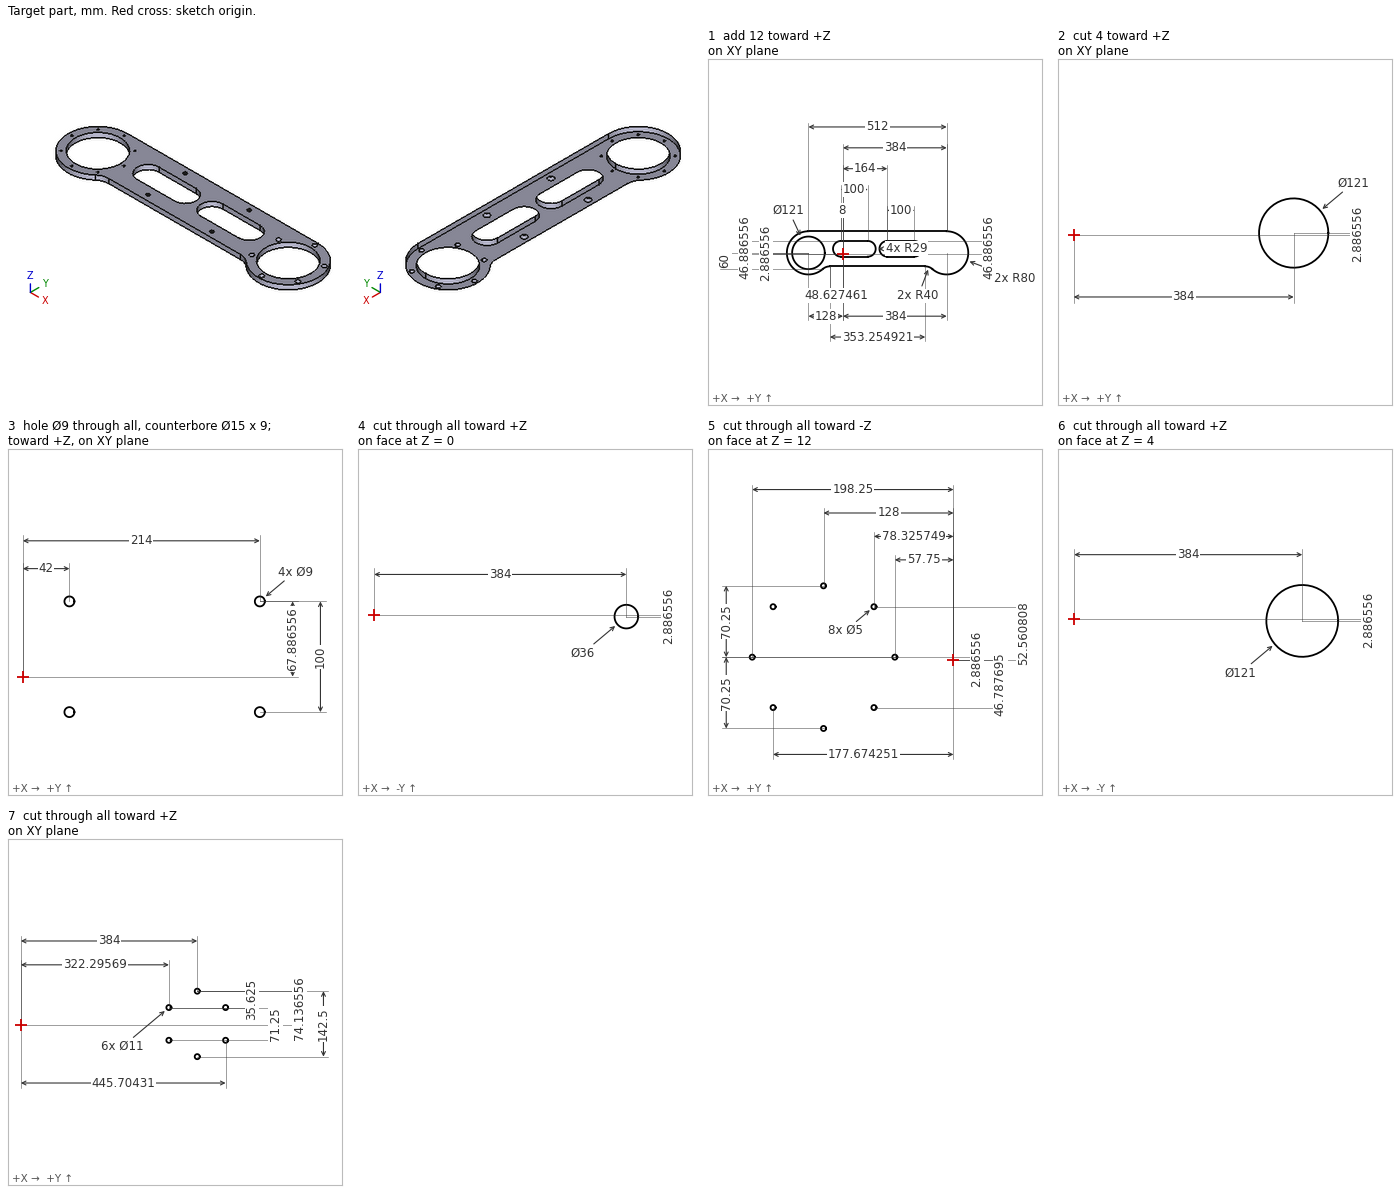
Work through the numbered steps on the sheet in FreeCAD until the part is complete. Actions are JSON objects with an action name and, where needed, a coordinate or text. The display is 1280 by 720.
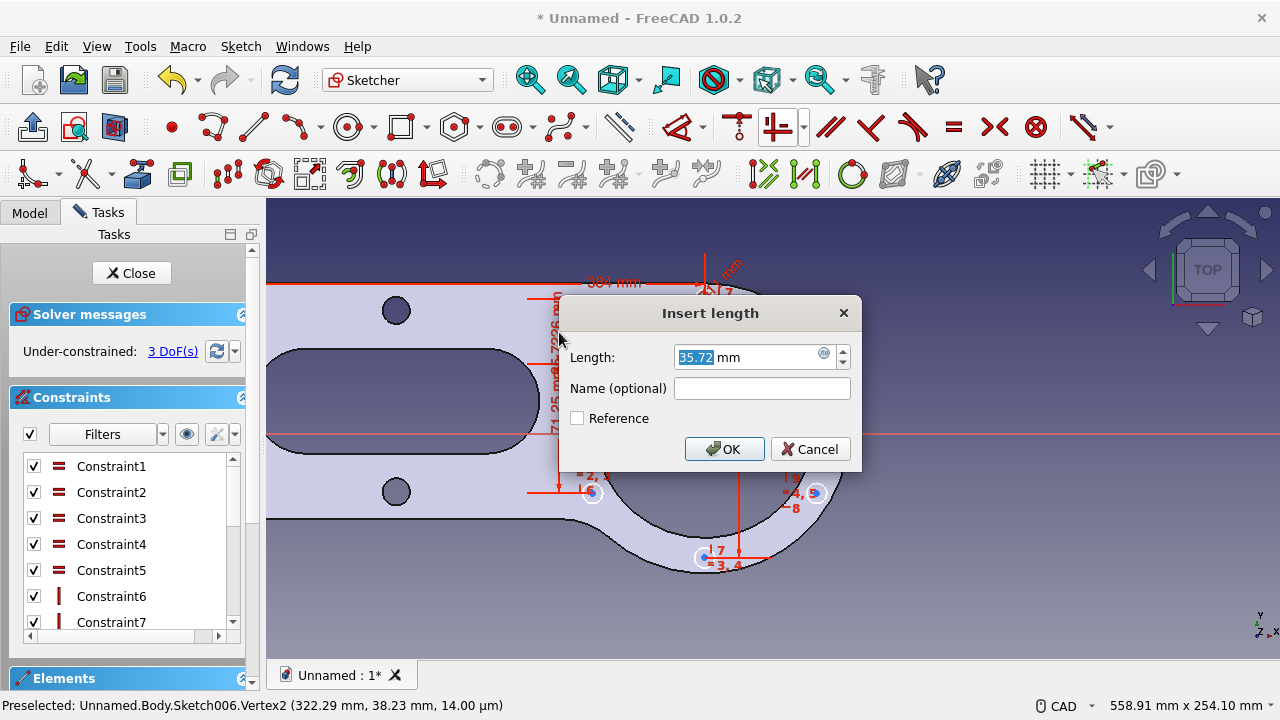
{"action": "type", "text": "35.625"}
{"action": "key", "text": "Return"}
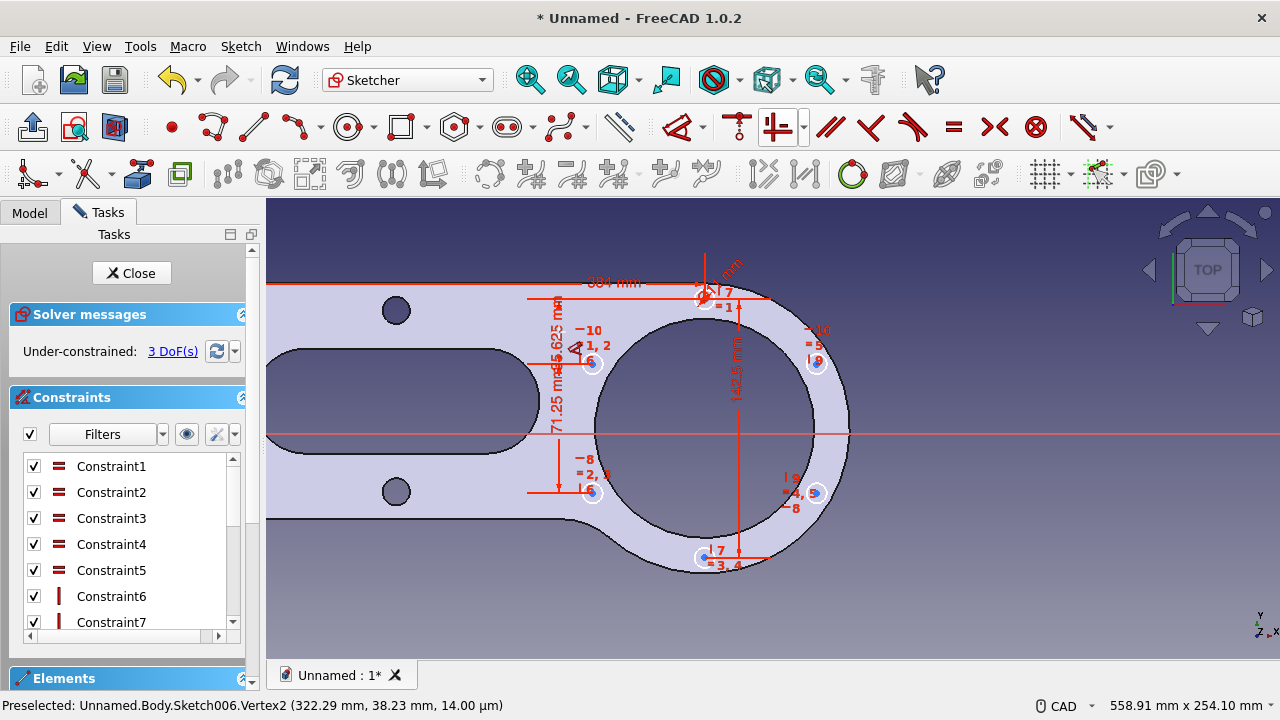
{"action": "left_click", "coordinate": [705, 299]}
{"action": "left_click", "coordinate": [739, 336]}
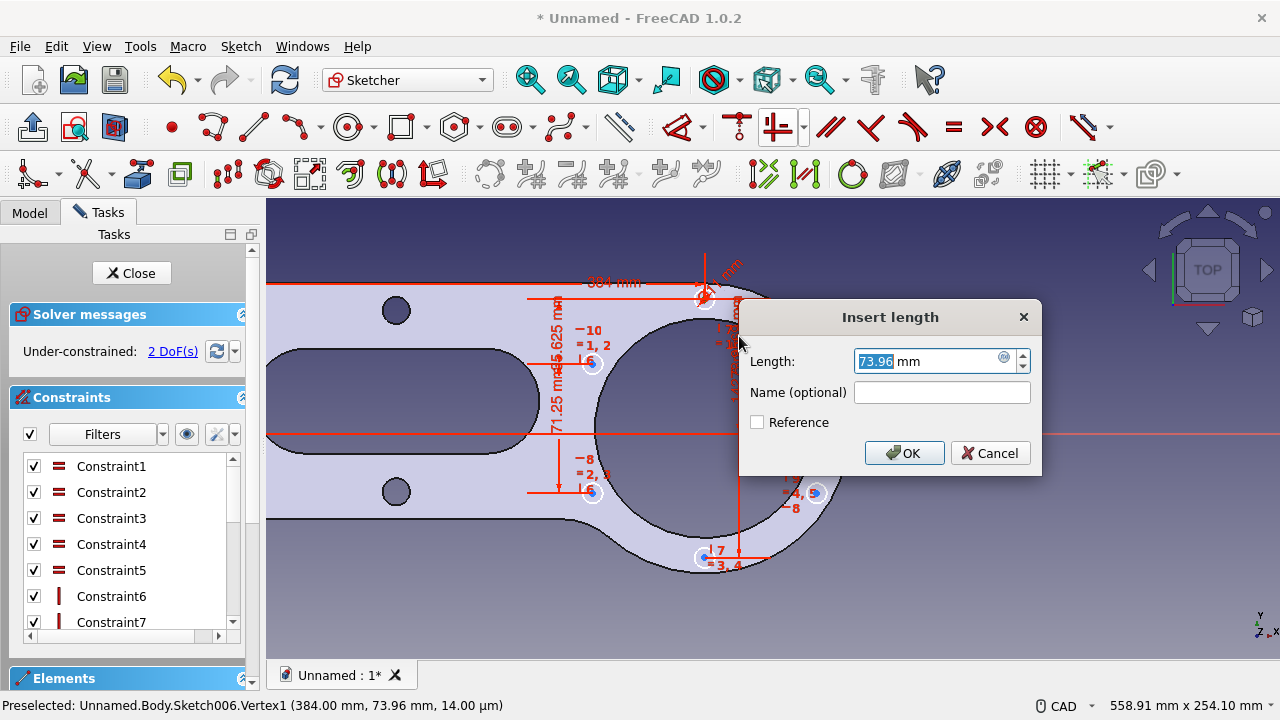
{"action": "type", "text": "74.136556"}
{"action": "key", "text": "Return"}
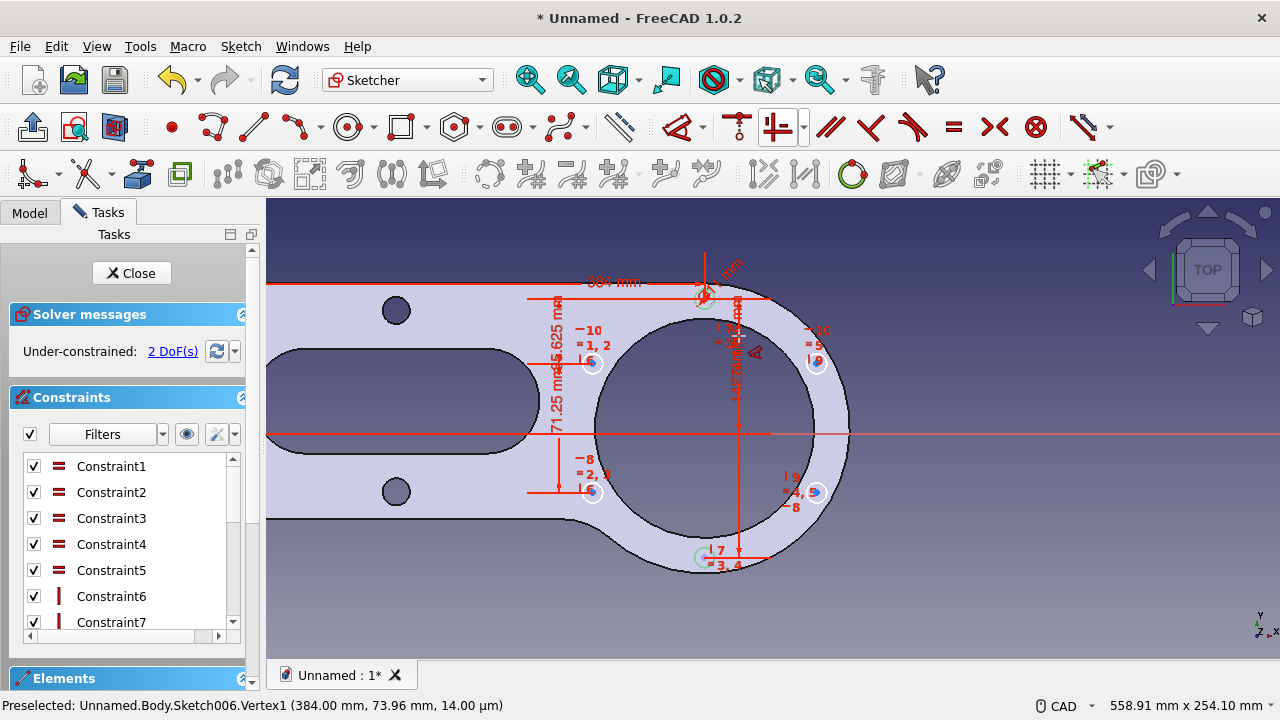
{"action": "left_click", "coordinate": [593, 364]}
{"action": "left_click", "coordinate": [443, 330]}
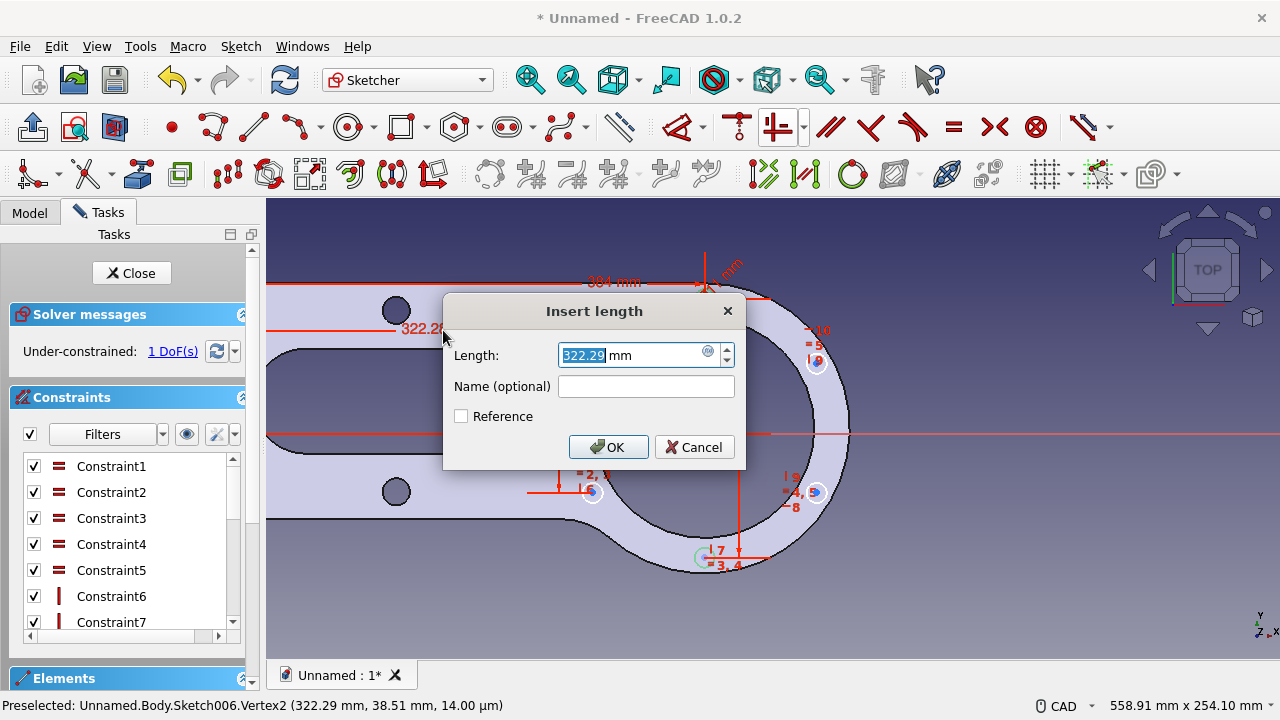
{"action": "type", "text": "322.29569"}
{"action": "key", "text": "Return"}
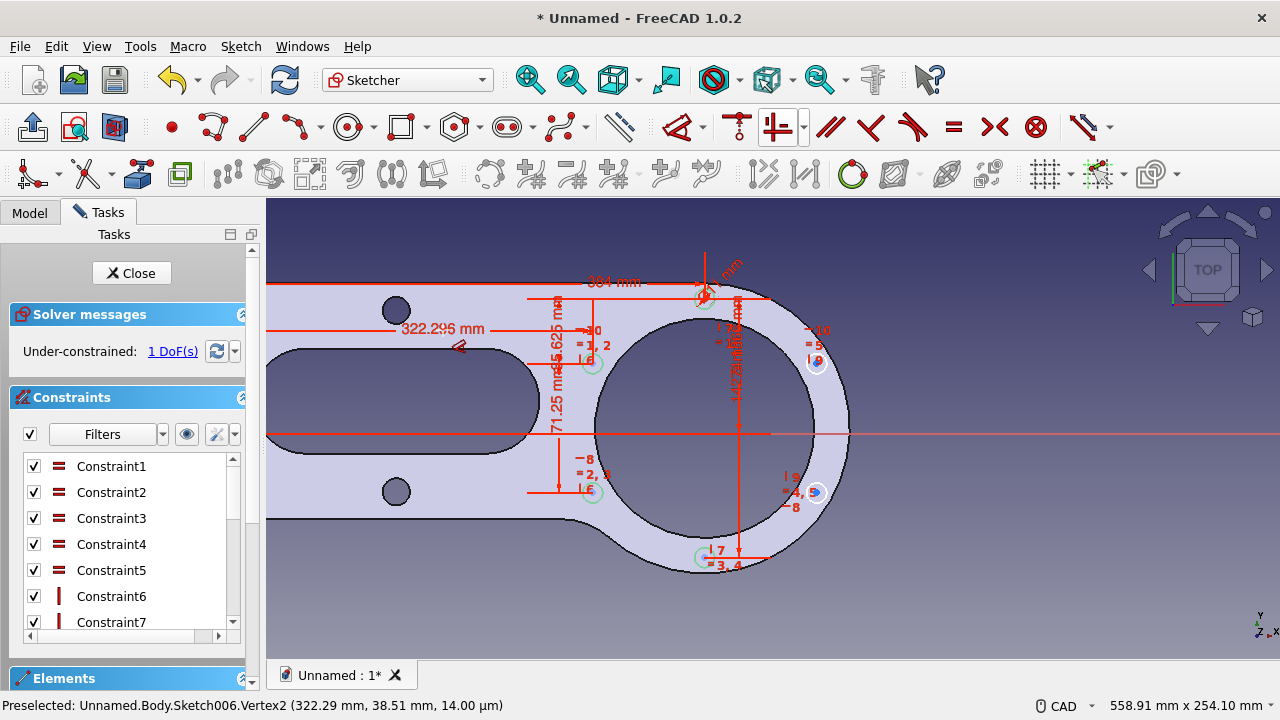
{"action": "left_click", "coordinate": [817, 493]}
{"action": "left_click", "coordinate": [555, 527]}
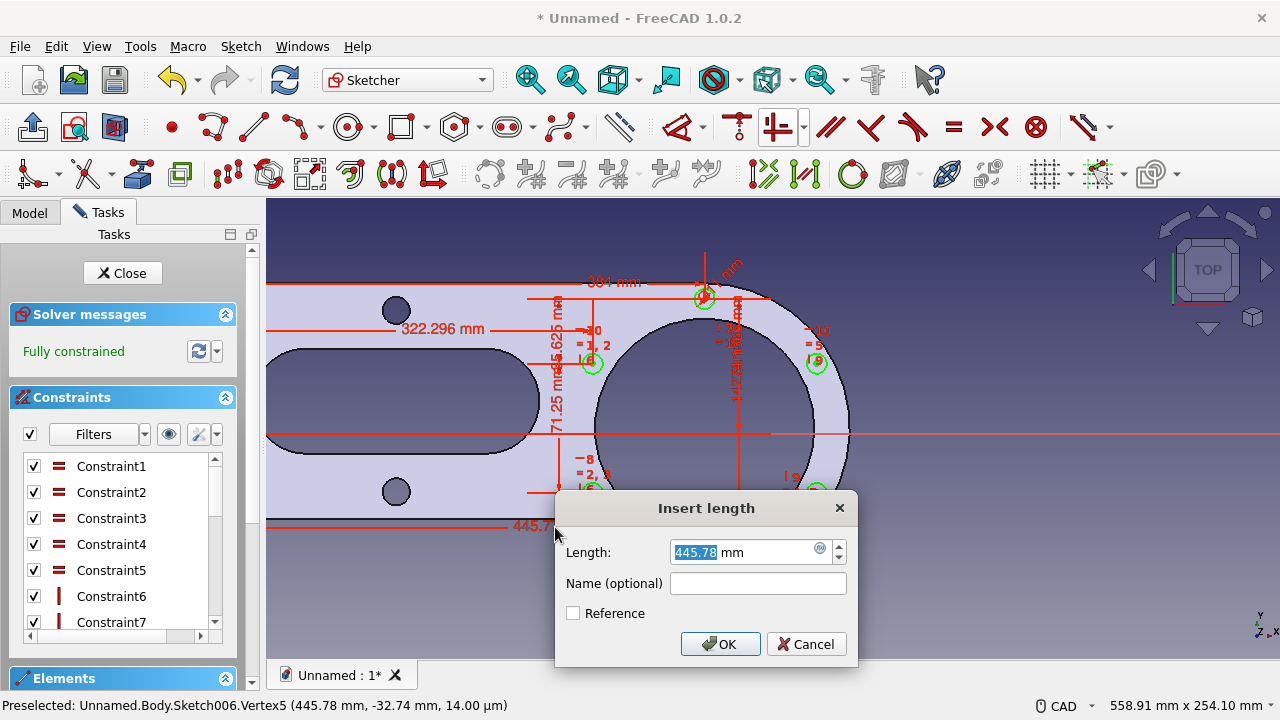
{"action": "type", "text": "445.70431"}
{"action": "key", "text": "Return"}
{"action": "key", "text": "Escape"}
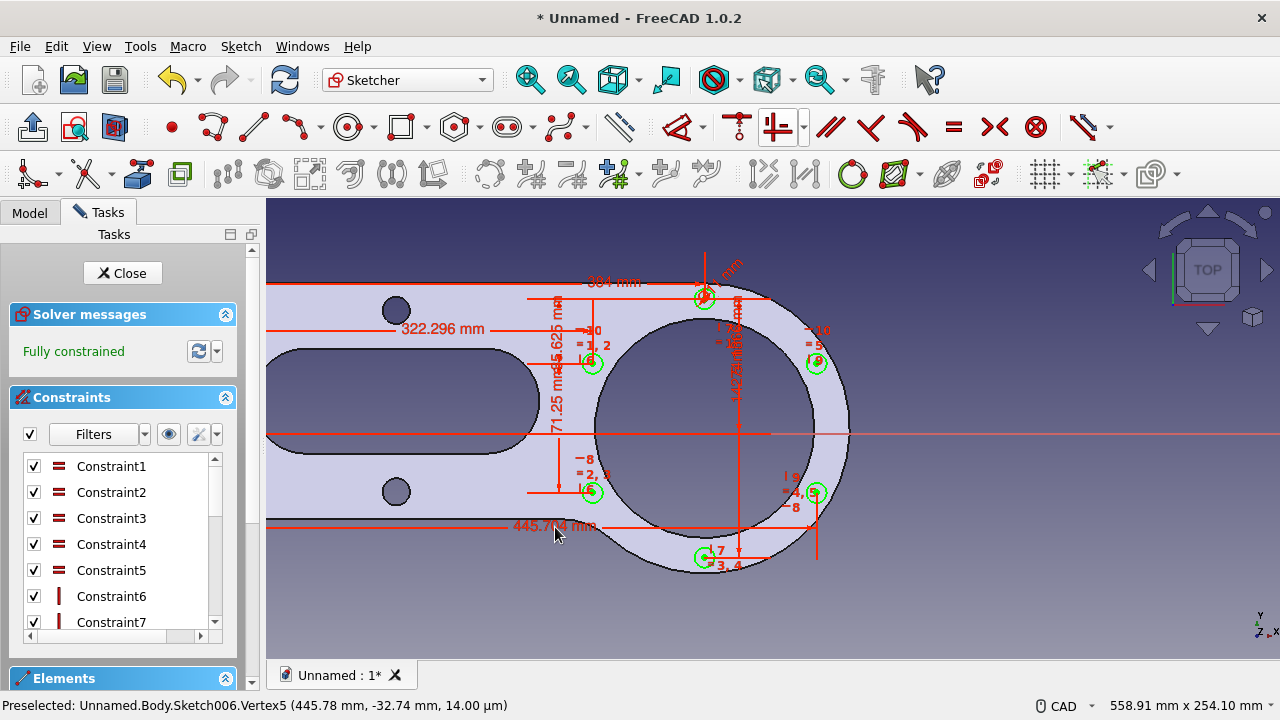
{"action": "left_click", "coordinate": [123, 273]}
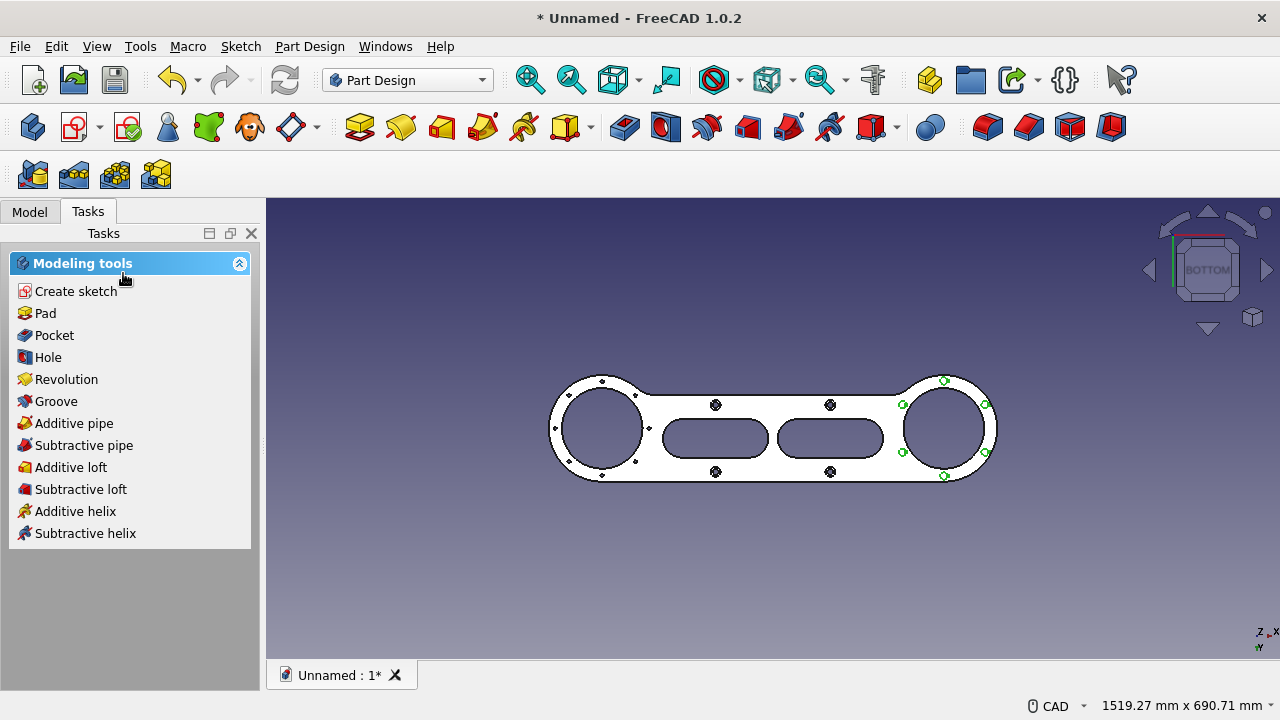
{"action": "left_click", "coordinate": [625, 128]}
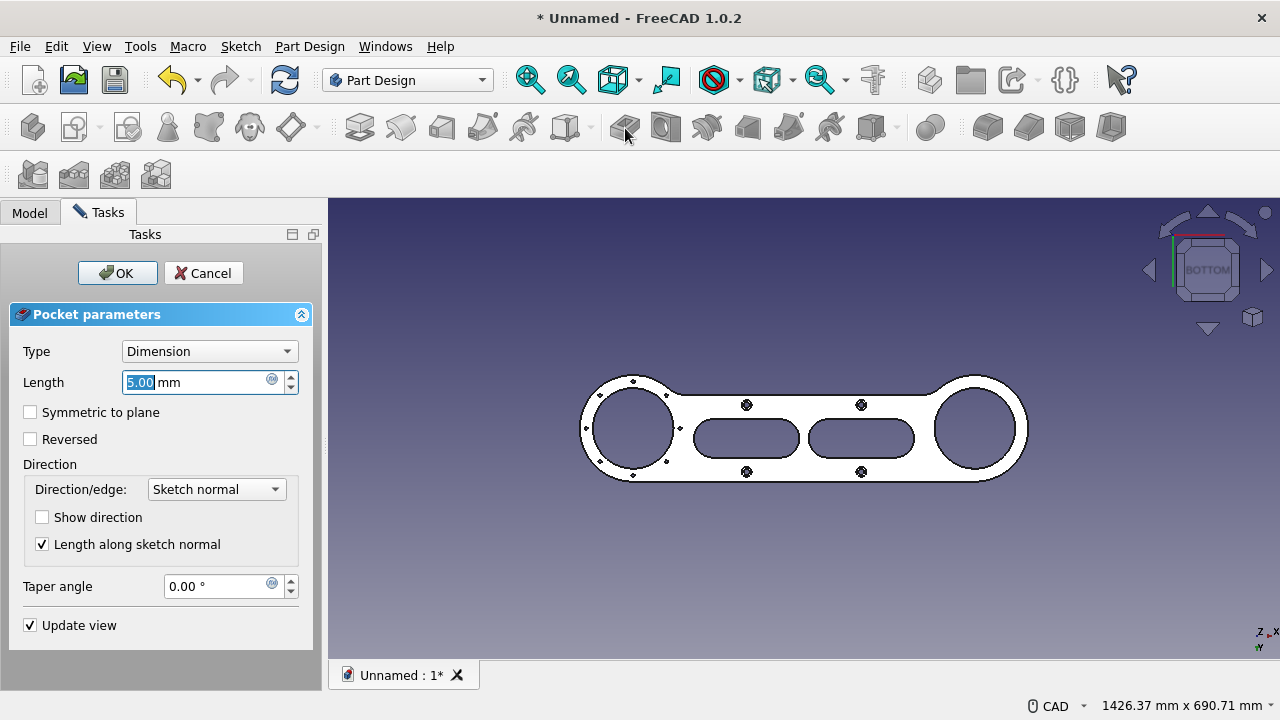
{"action": "left_click", "coordinate": [210, 352]}